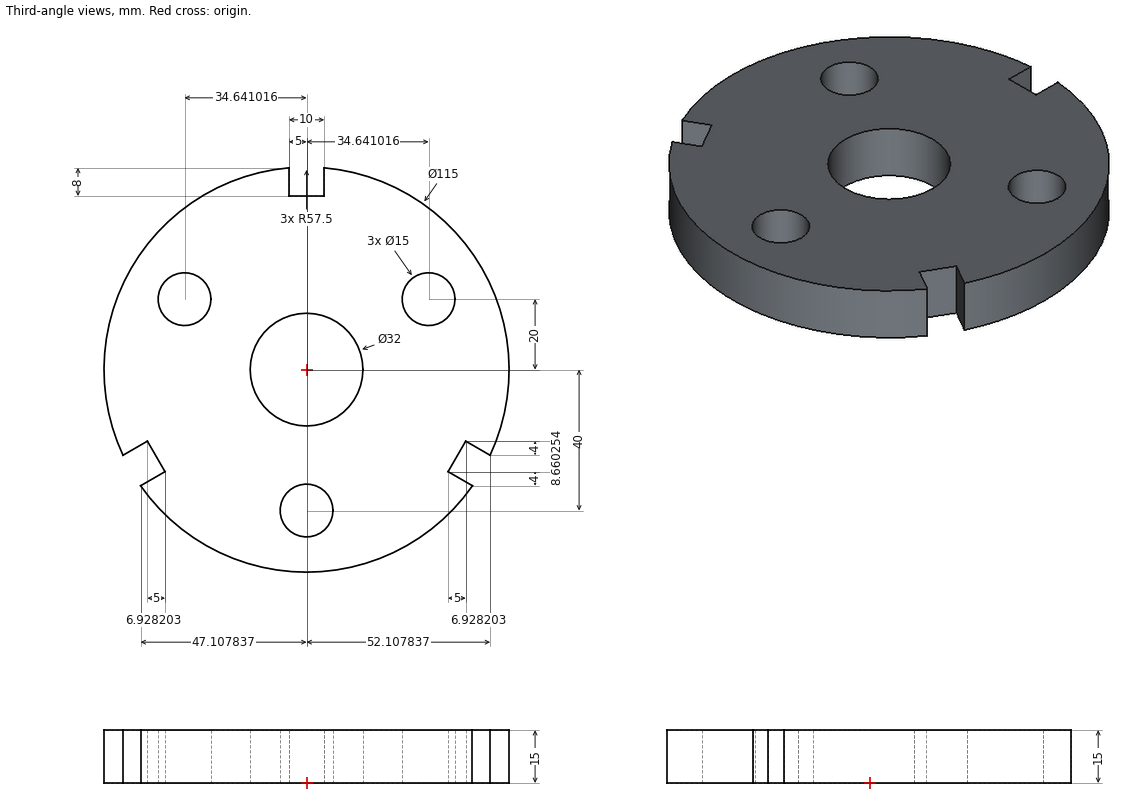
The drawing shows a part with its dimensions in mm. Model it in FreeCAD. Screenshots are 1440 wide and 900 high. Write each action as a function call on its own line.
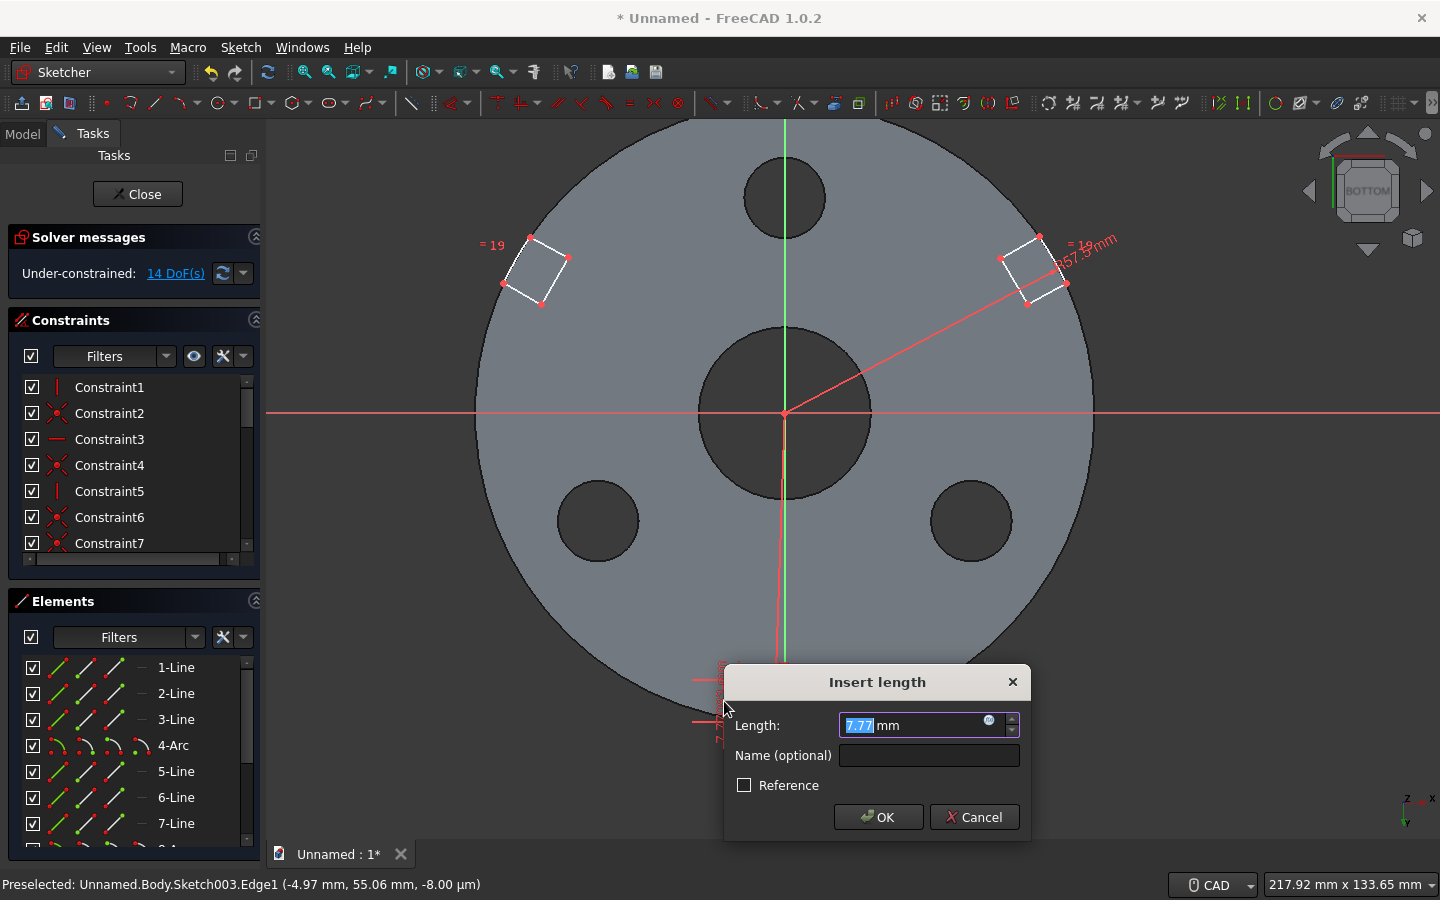
text(8)
key(Return)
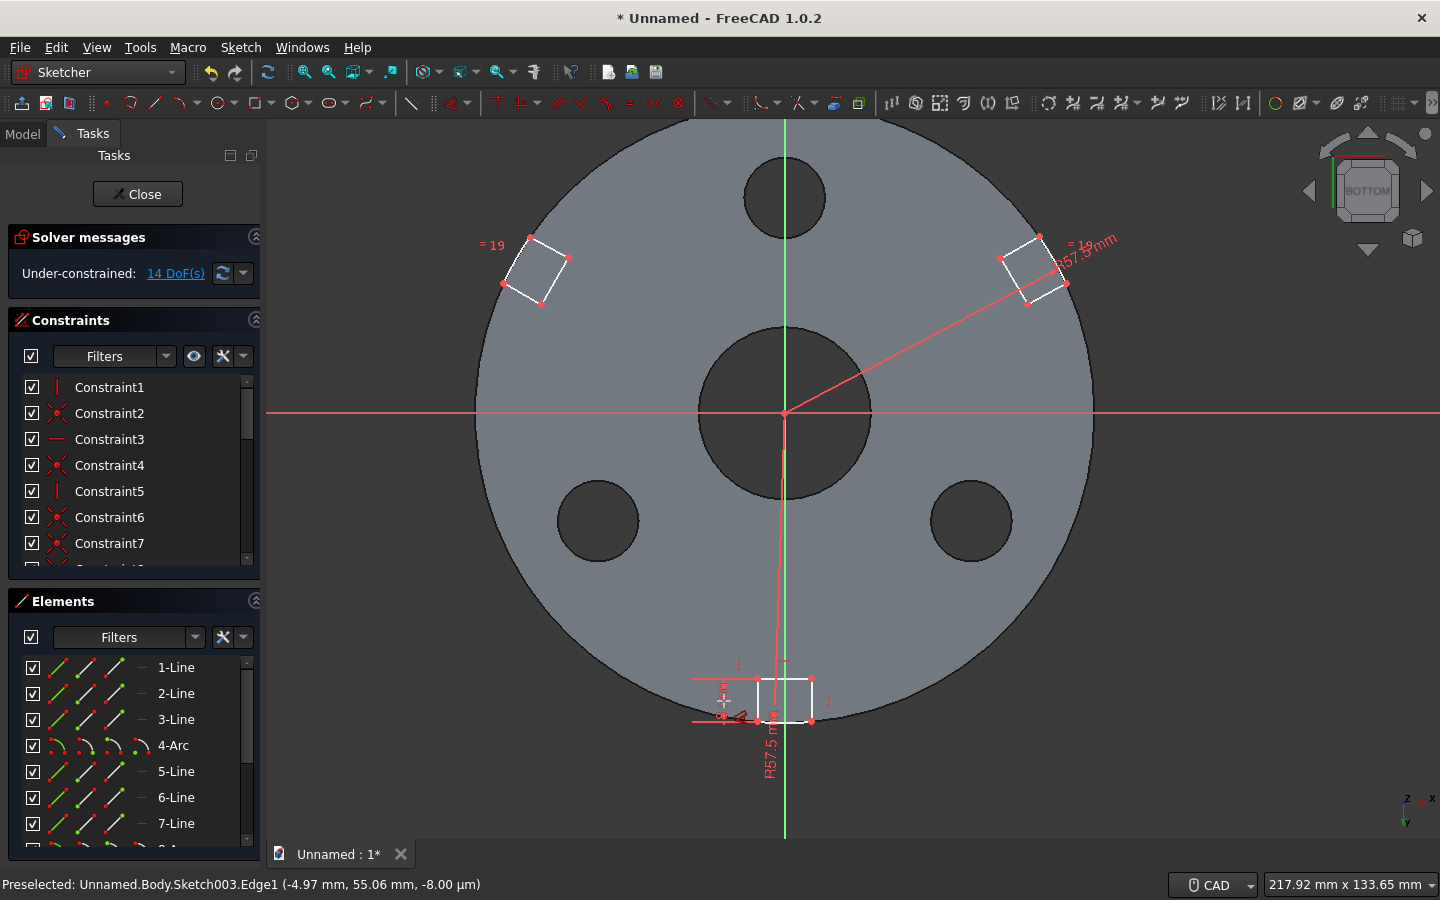
scroll(774, 679, up, 2)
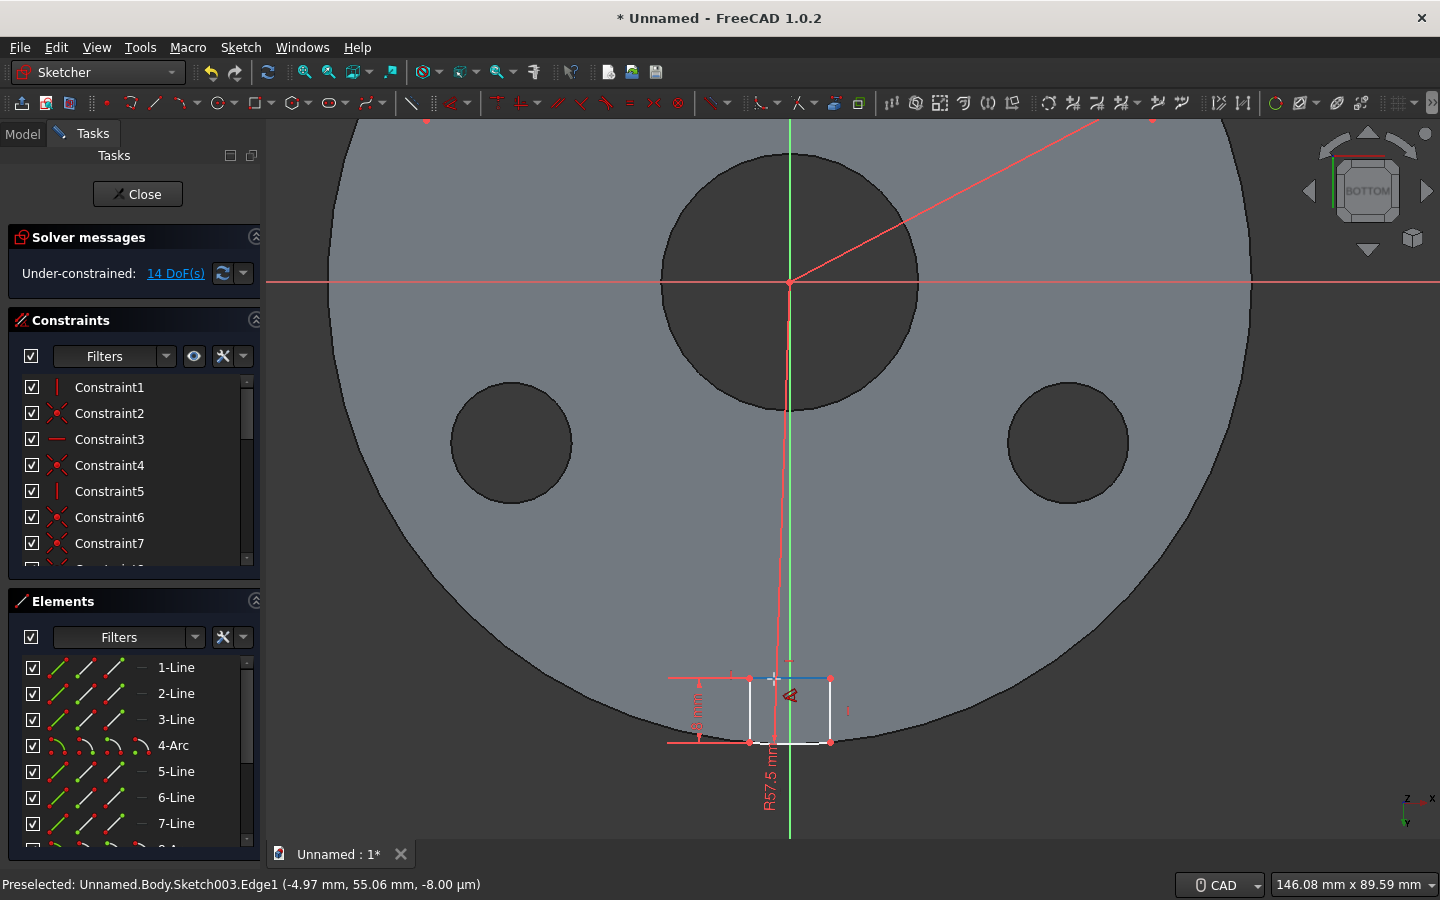
click(774, 678)
click(772, 712)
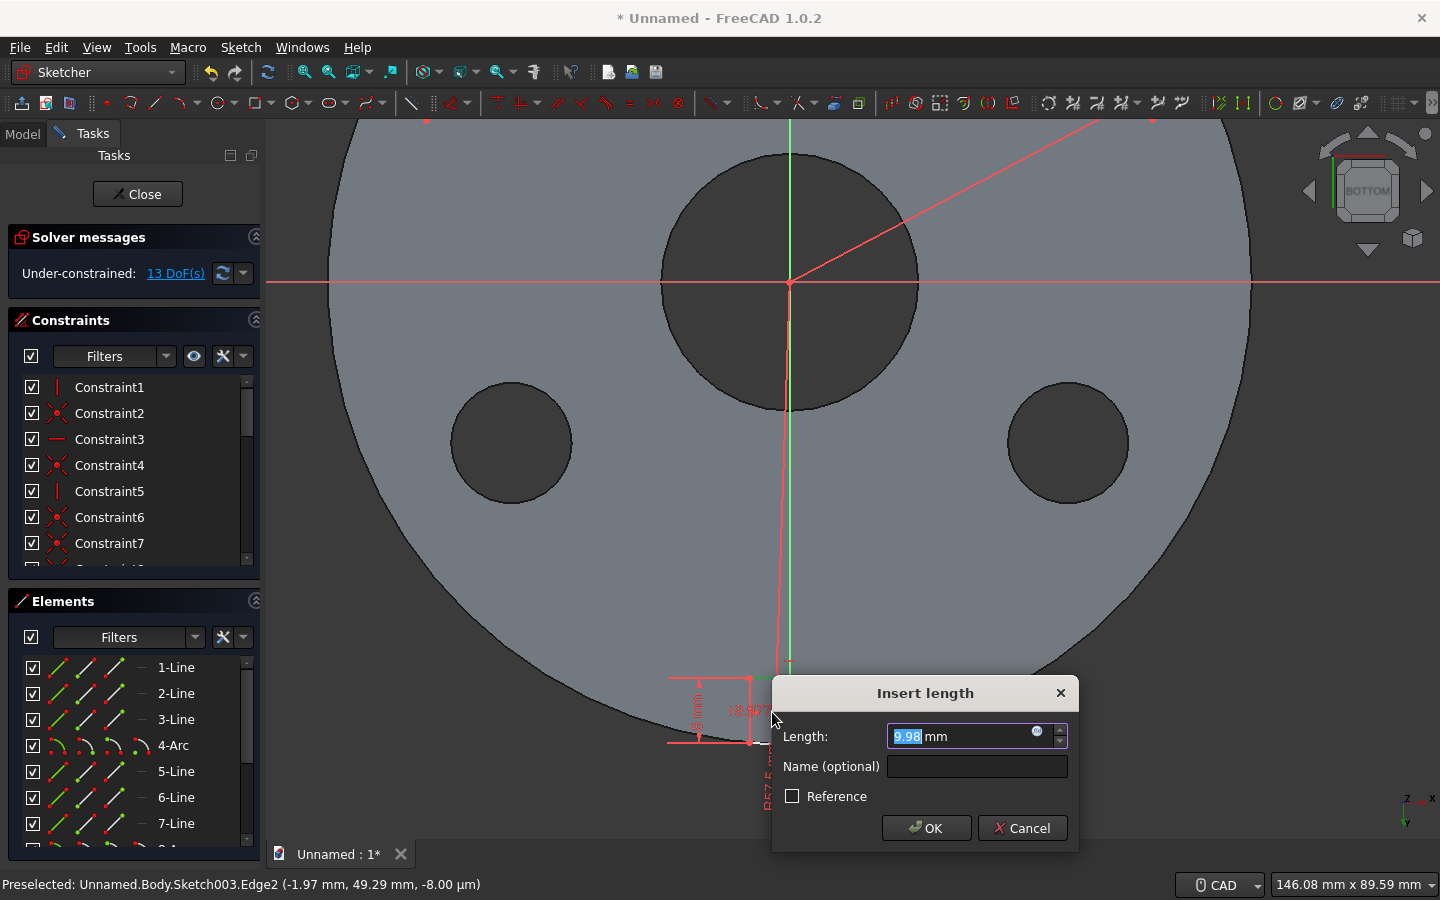
text(10)
key(Return)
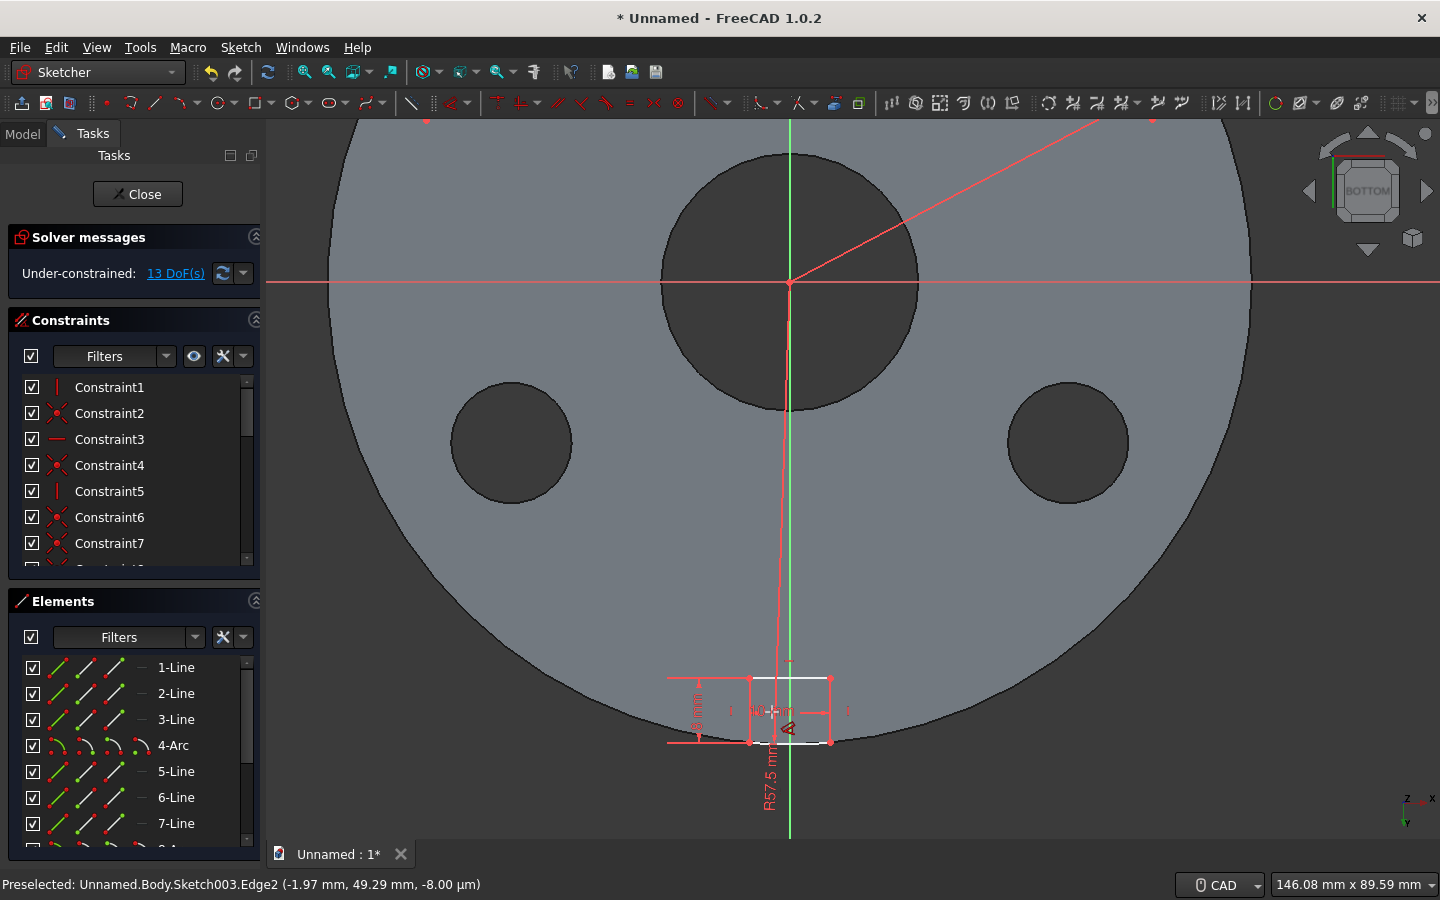
click(750, 743)
click(770, 248)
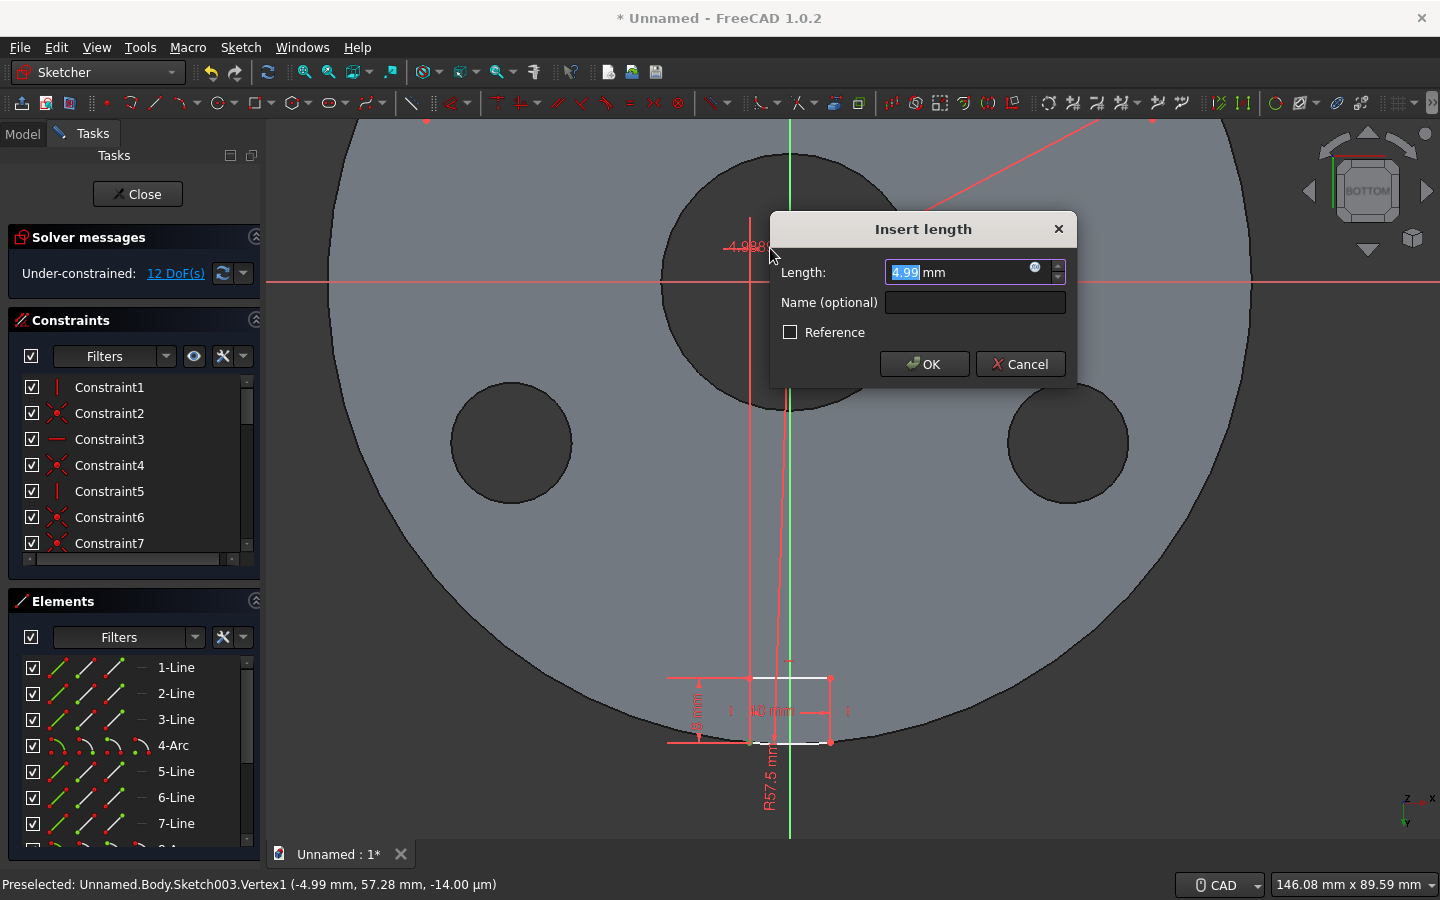
text(5)
key(Return)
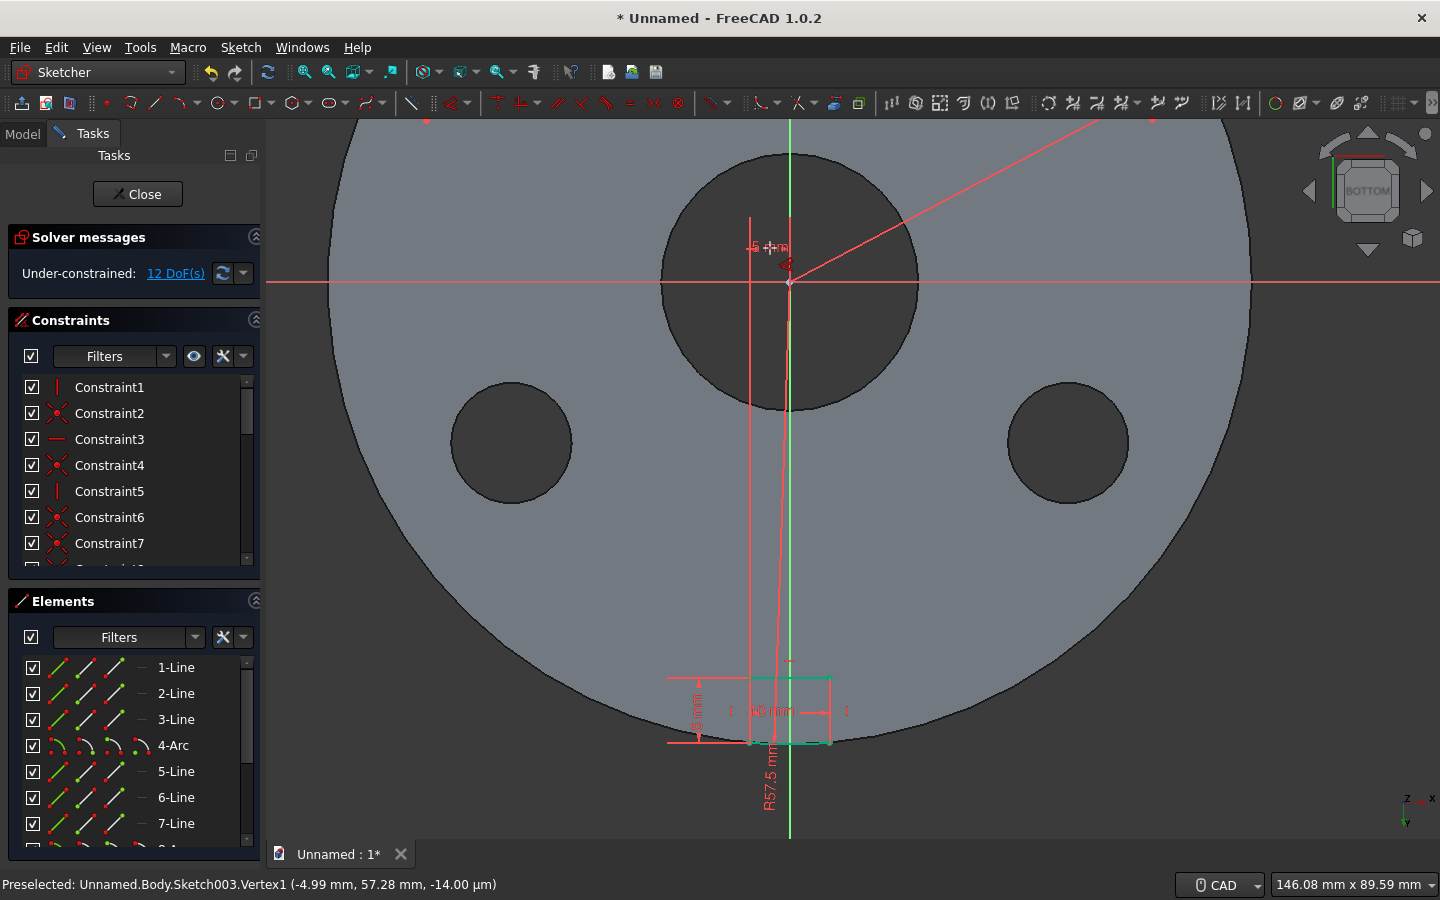
scroll(774, 678, down, 2)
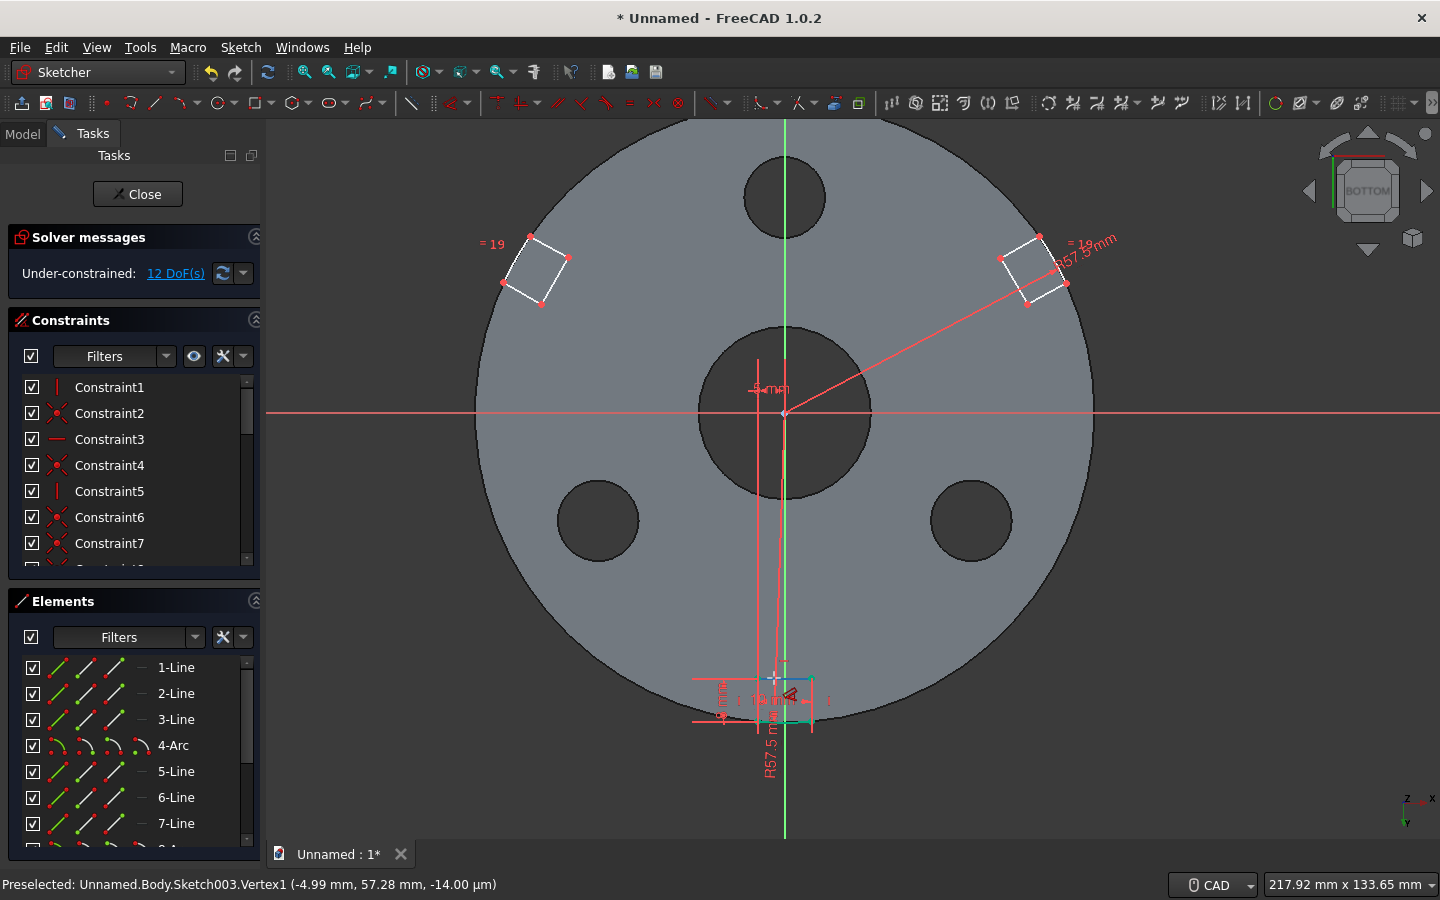
scroll(1055, 290, up, 4)